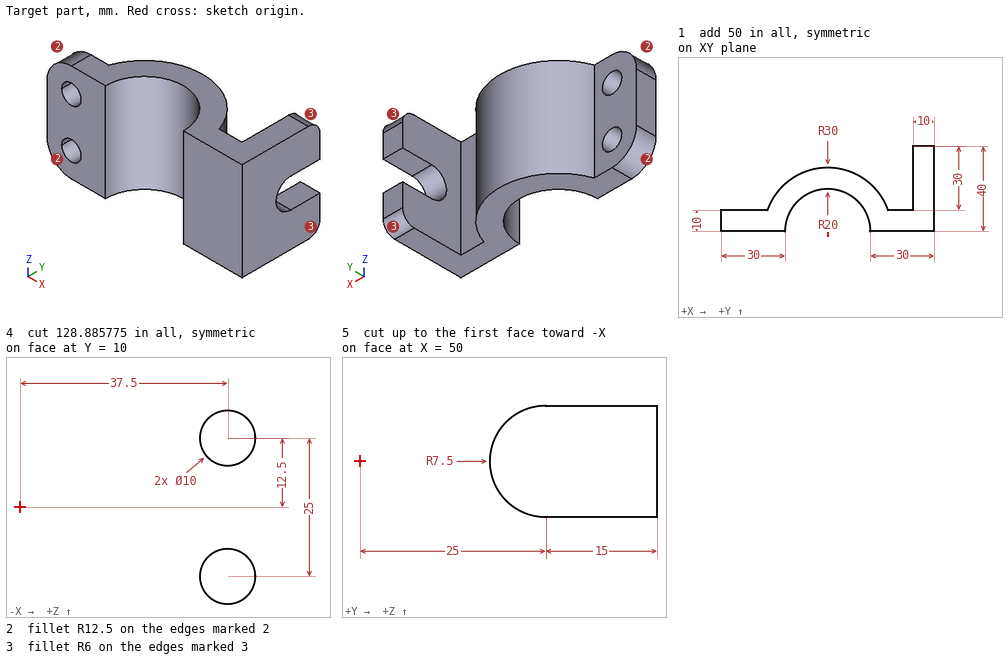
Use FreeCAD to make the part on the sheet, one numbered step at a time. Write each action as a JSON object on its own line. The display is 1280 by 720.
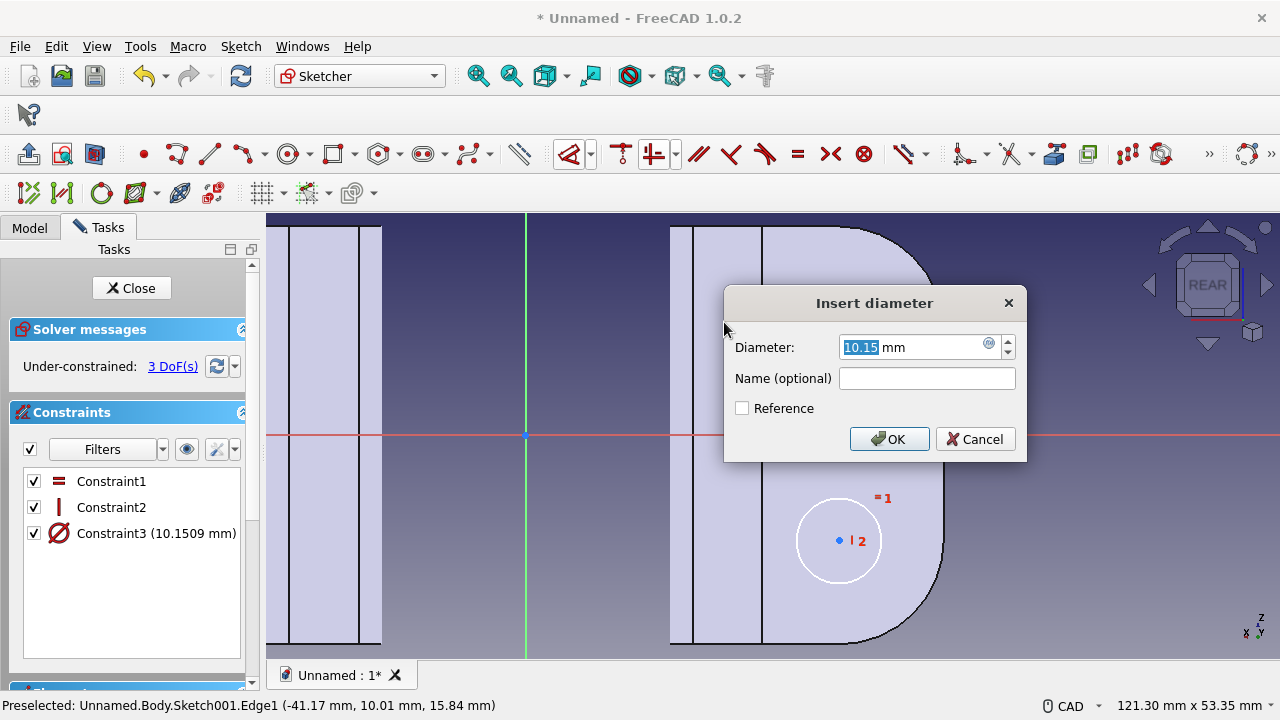
{"action": "type", "text": "10"}
{"action": "key", "text": "Return"}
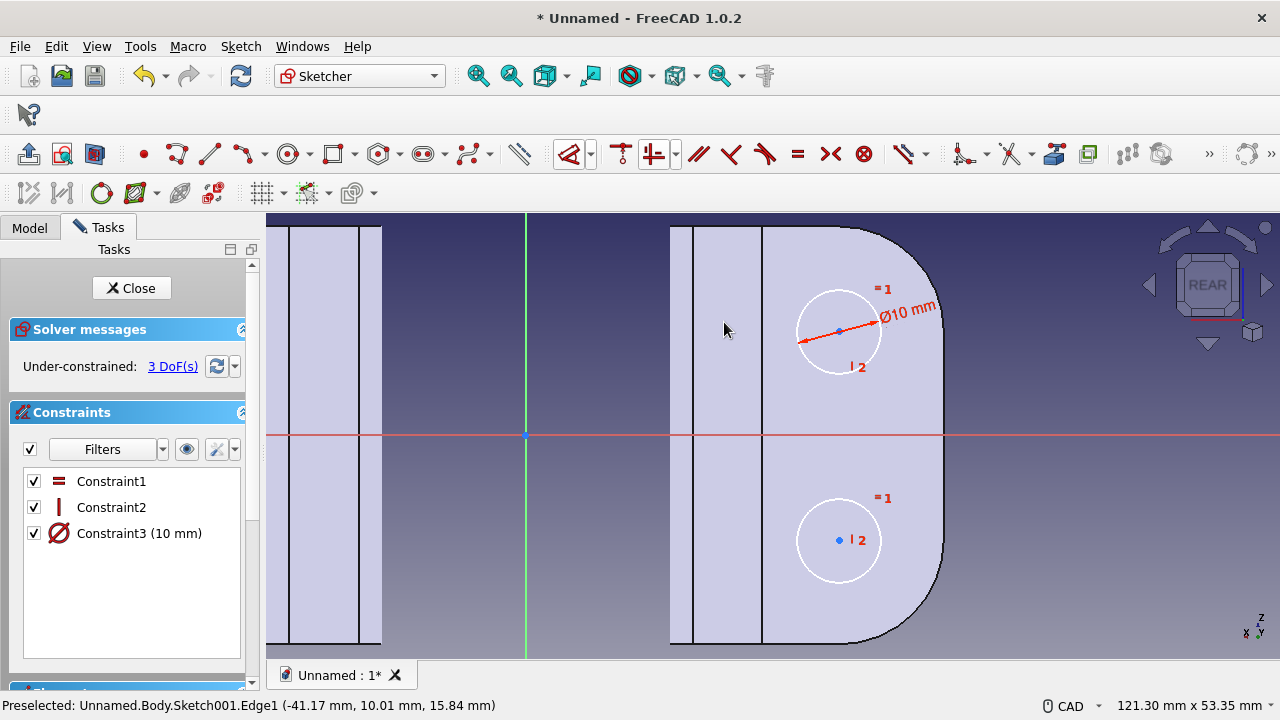
{"action": "left_click", "coordinate": [839, 332]}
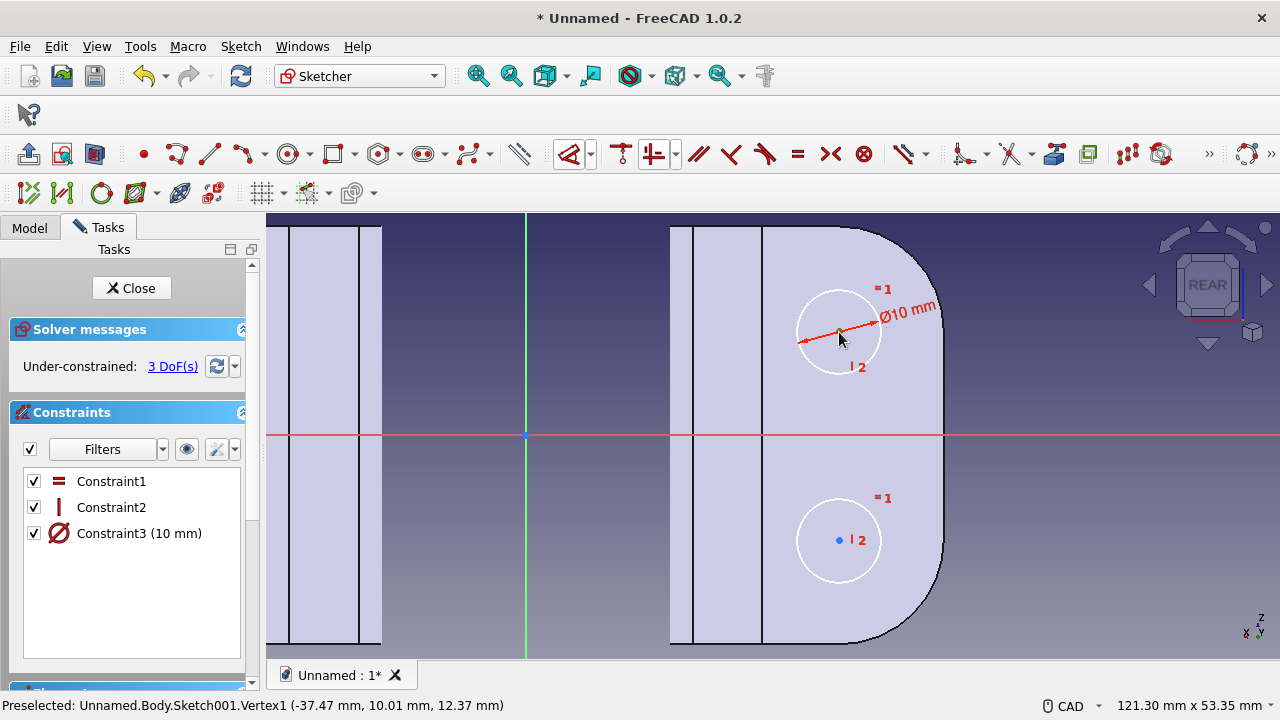
{"action": "left_click", "coordinate": [839, 541]}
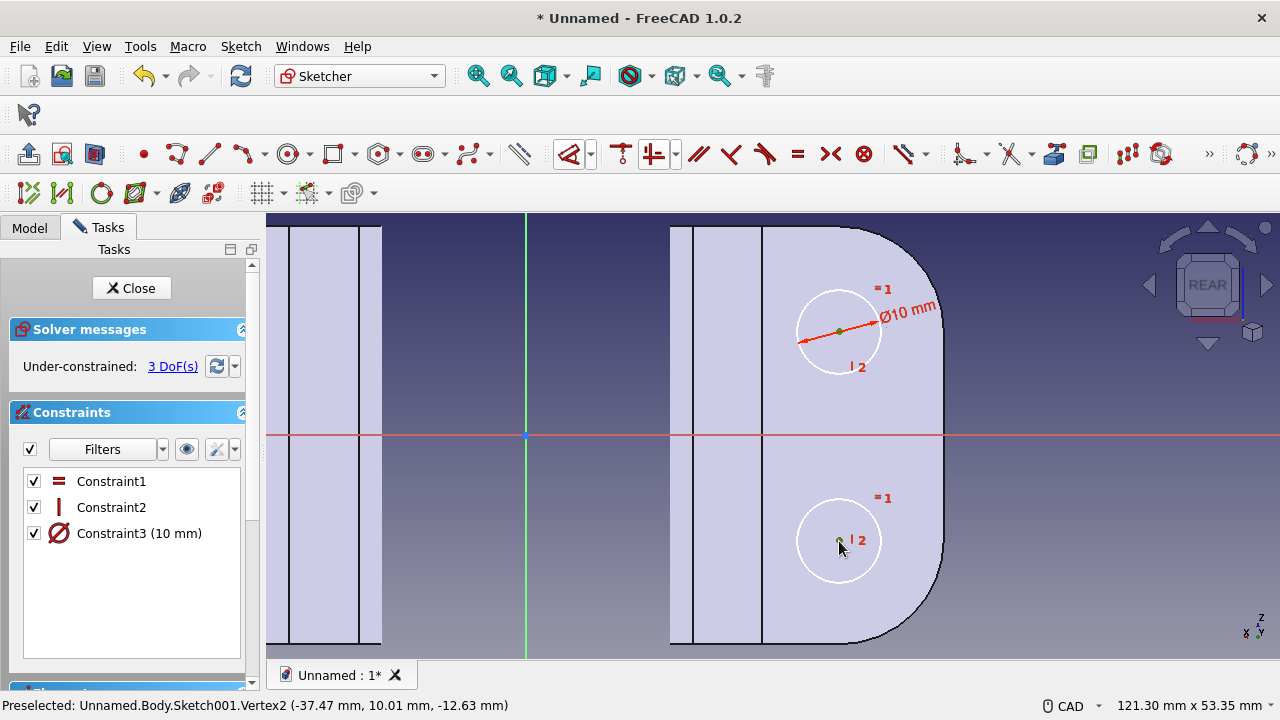
{"action": "left_click", "coordinate": [590, 154]}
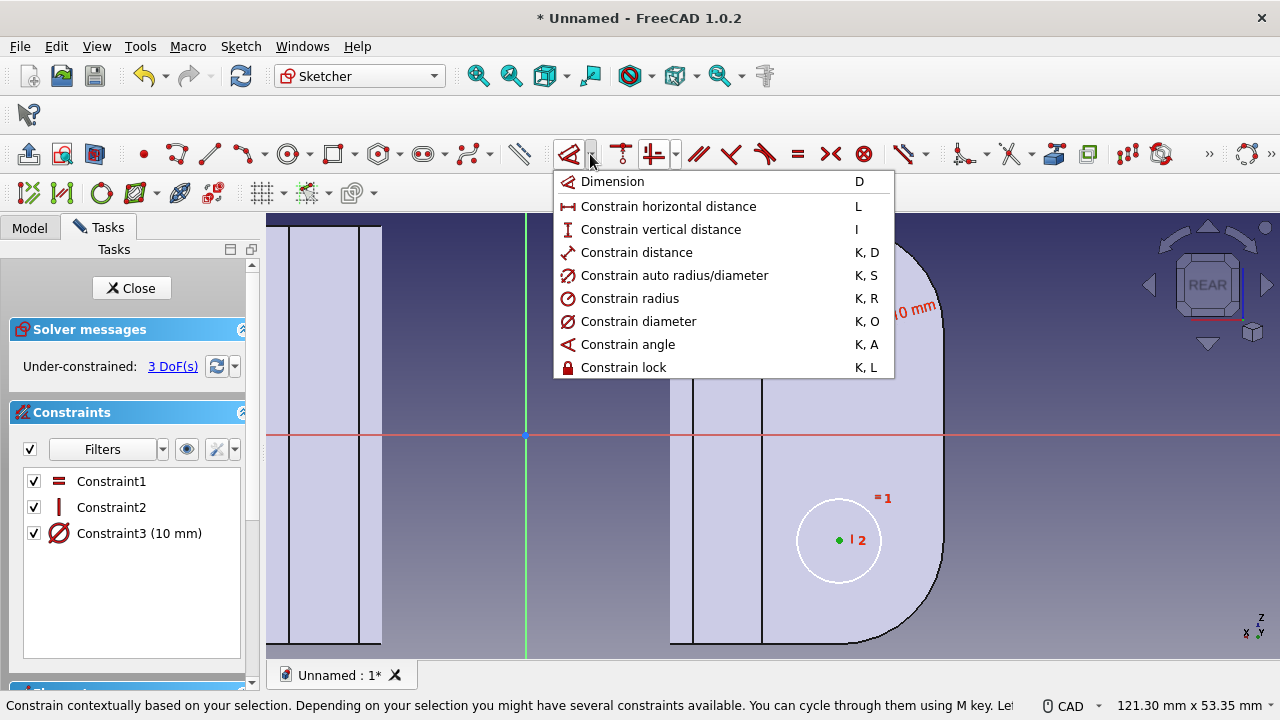
{"action": "left_click", "coordinate": [724, 230]}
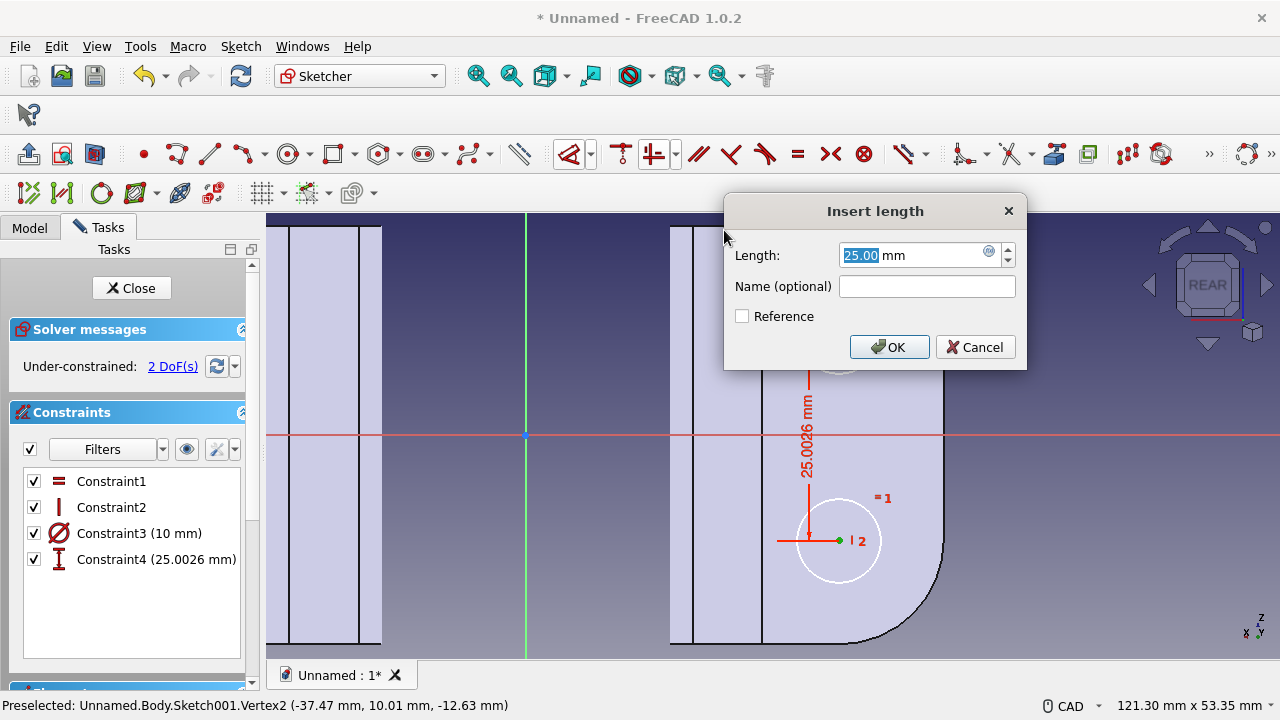
{"action": "type", "text": "25"}
{"action": "key", "text": "Return"}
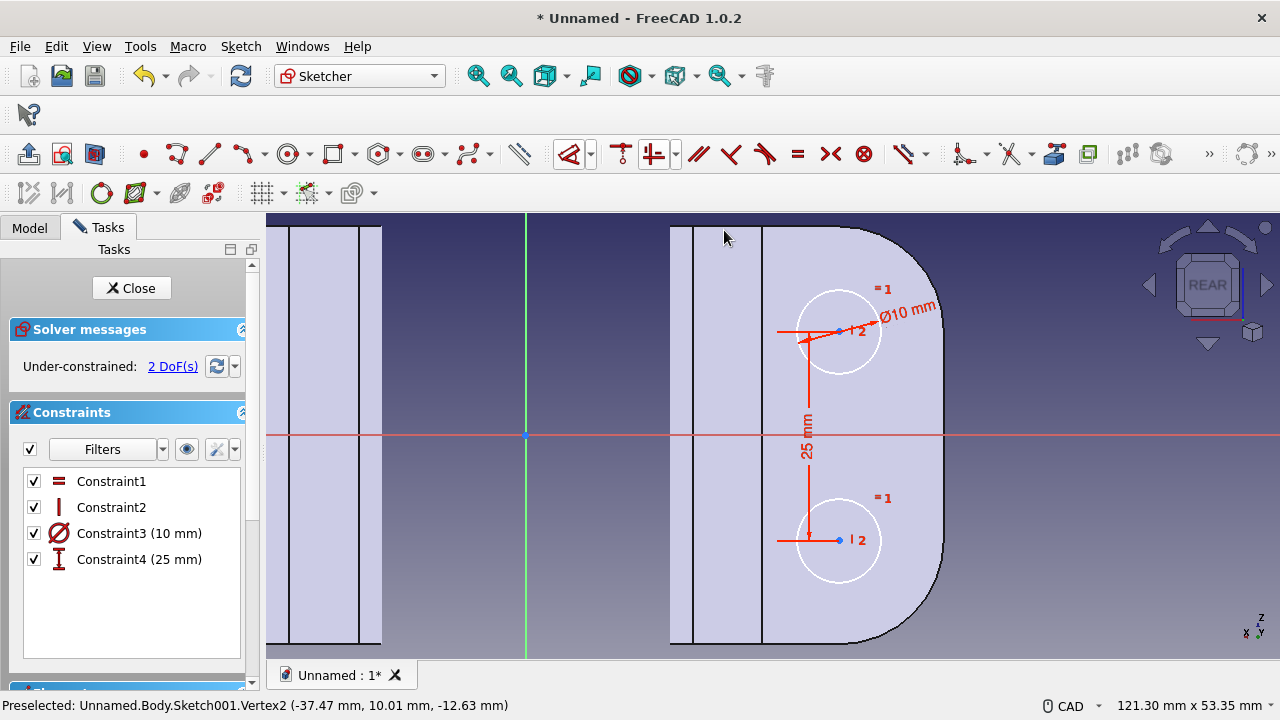
{"action": "left_click", "coordinate": [839, 332]}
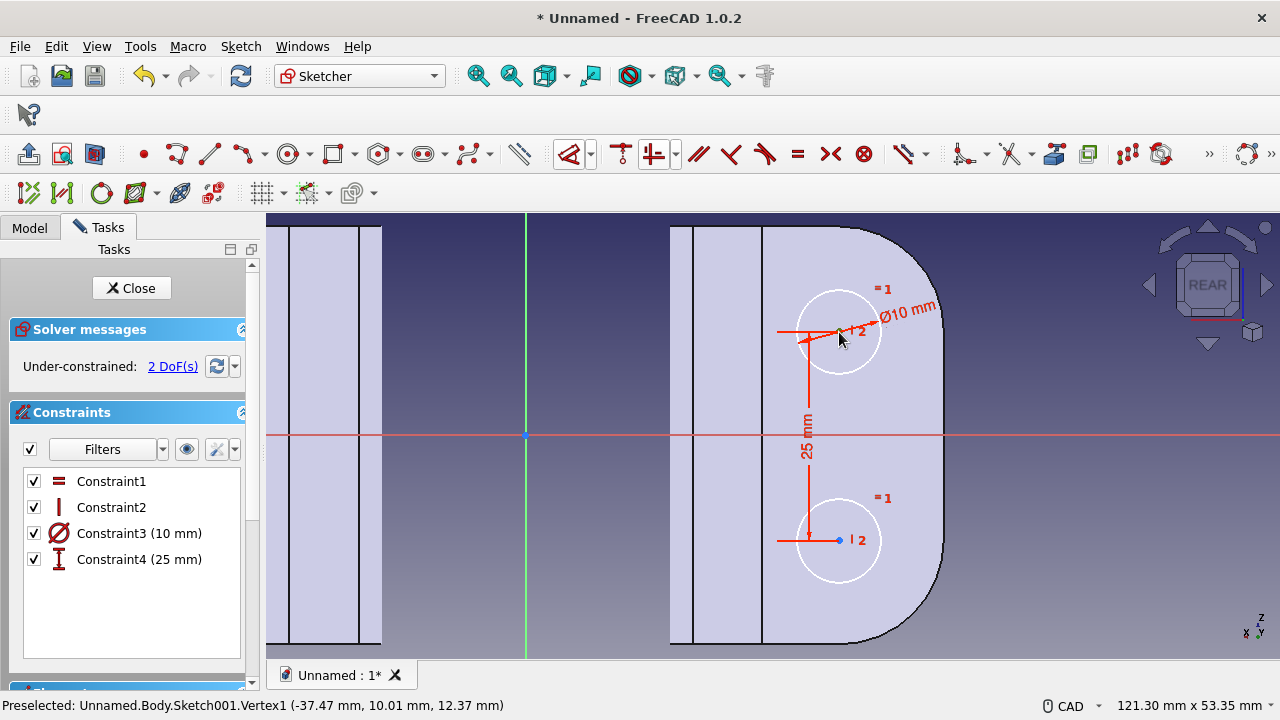
{"action": "left_click", "coordinate": [590, 154]}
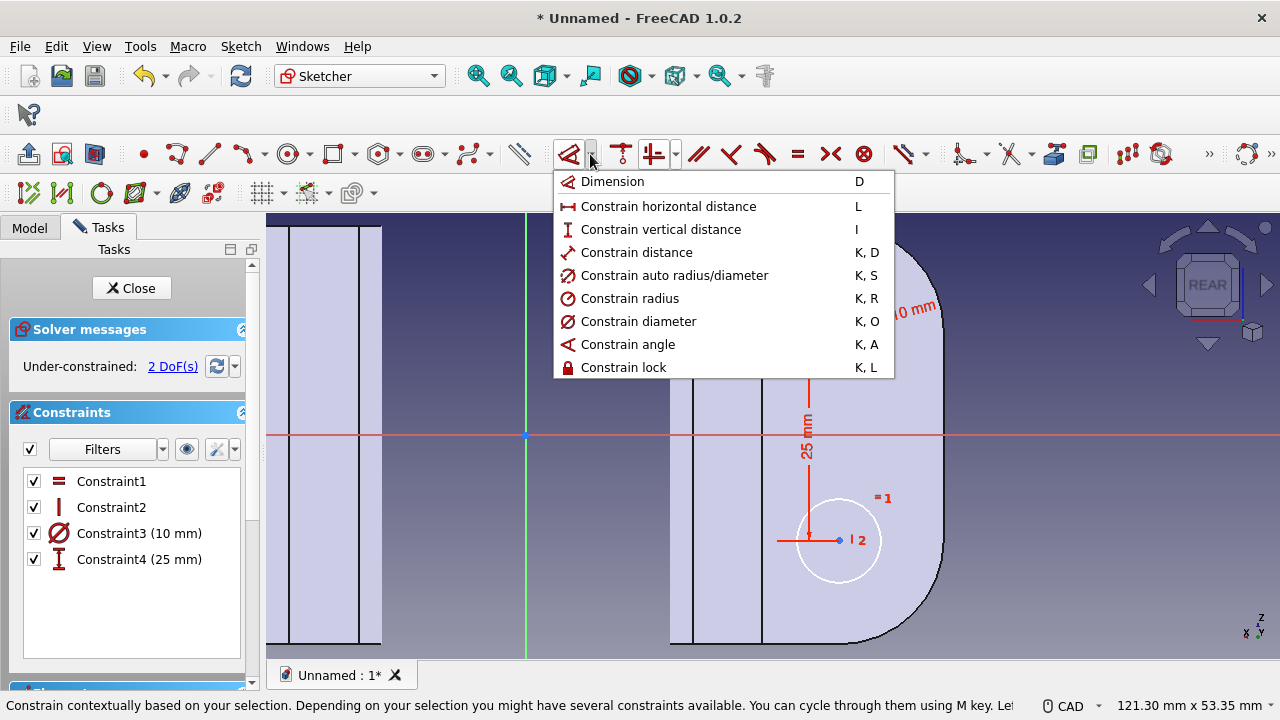
{"action": "left_click", "coordinate": [724, 206]}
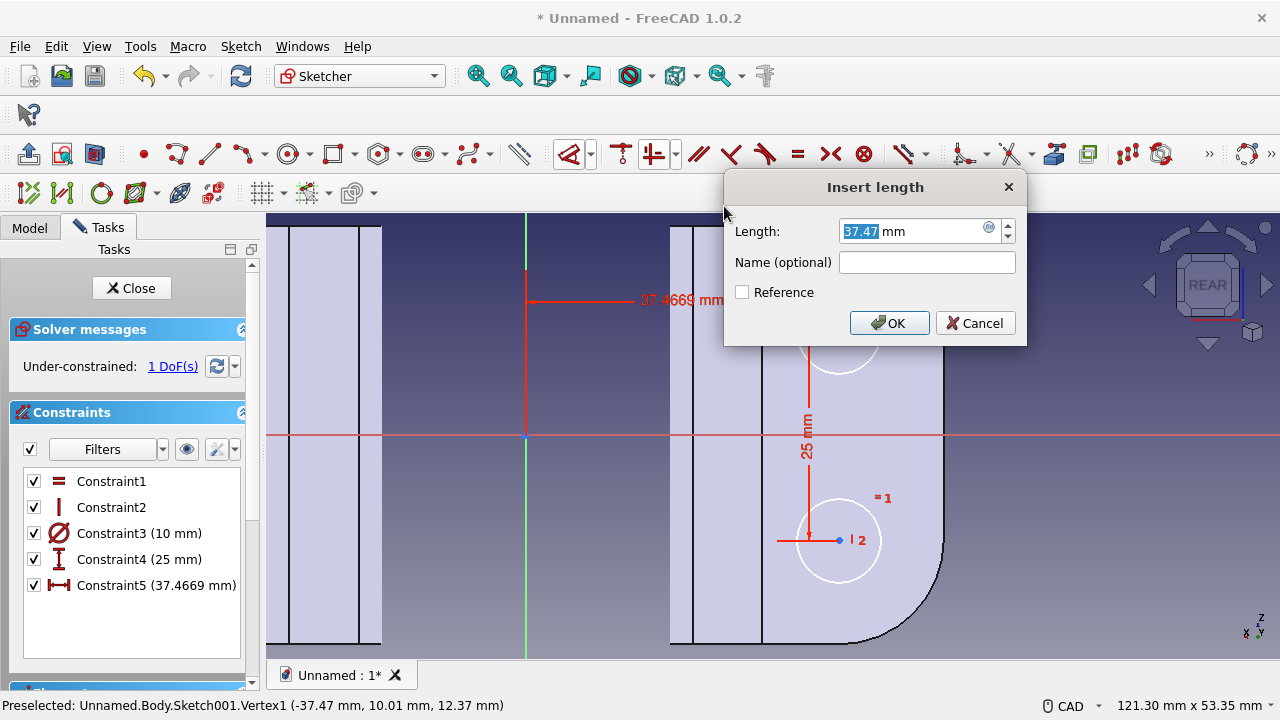
{"action": "type", "text": "37.5"}
{"action": "key", "text": "Return"}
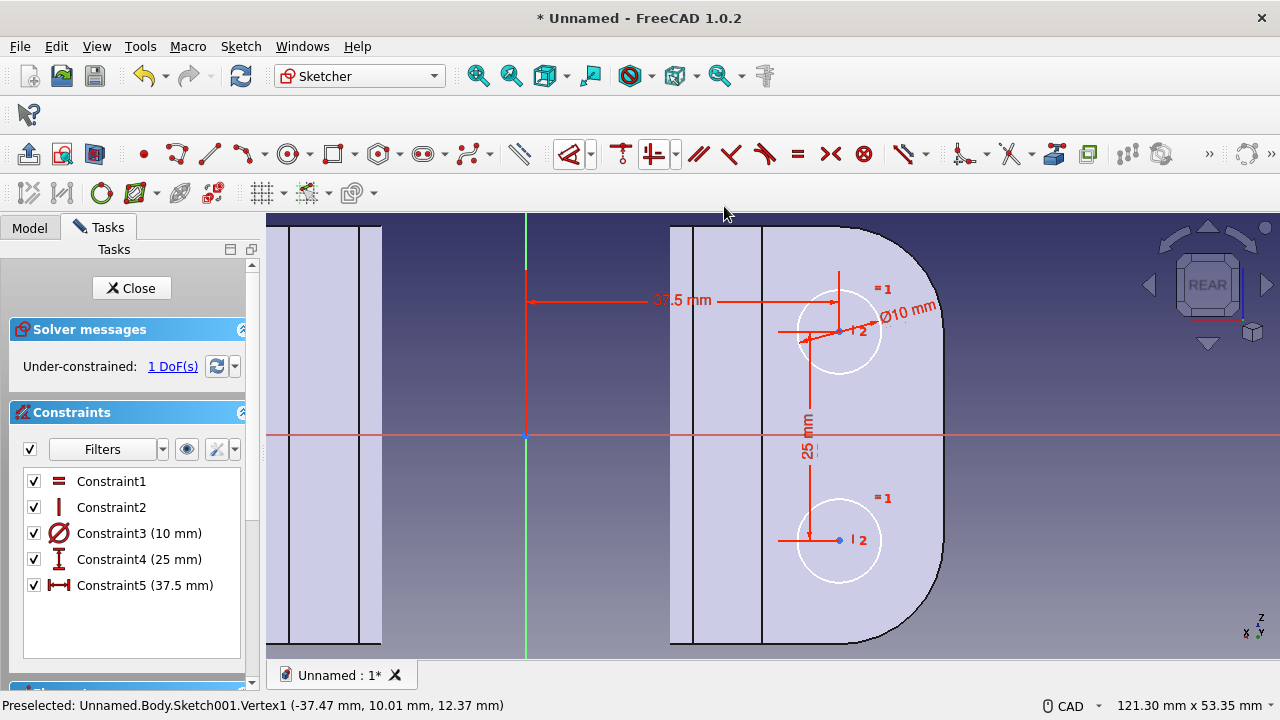
{"action": "left_click", "coordinate": [839, 332]}